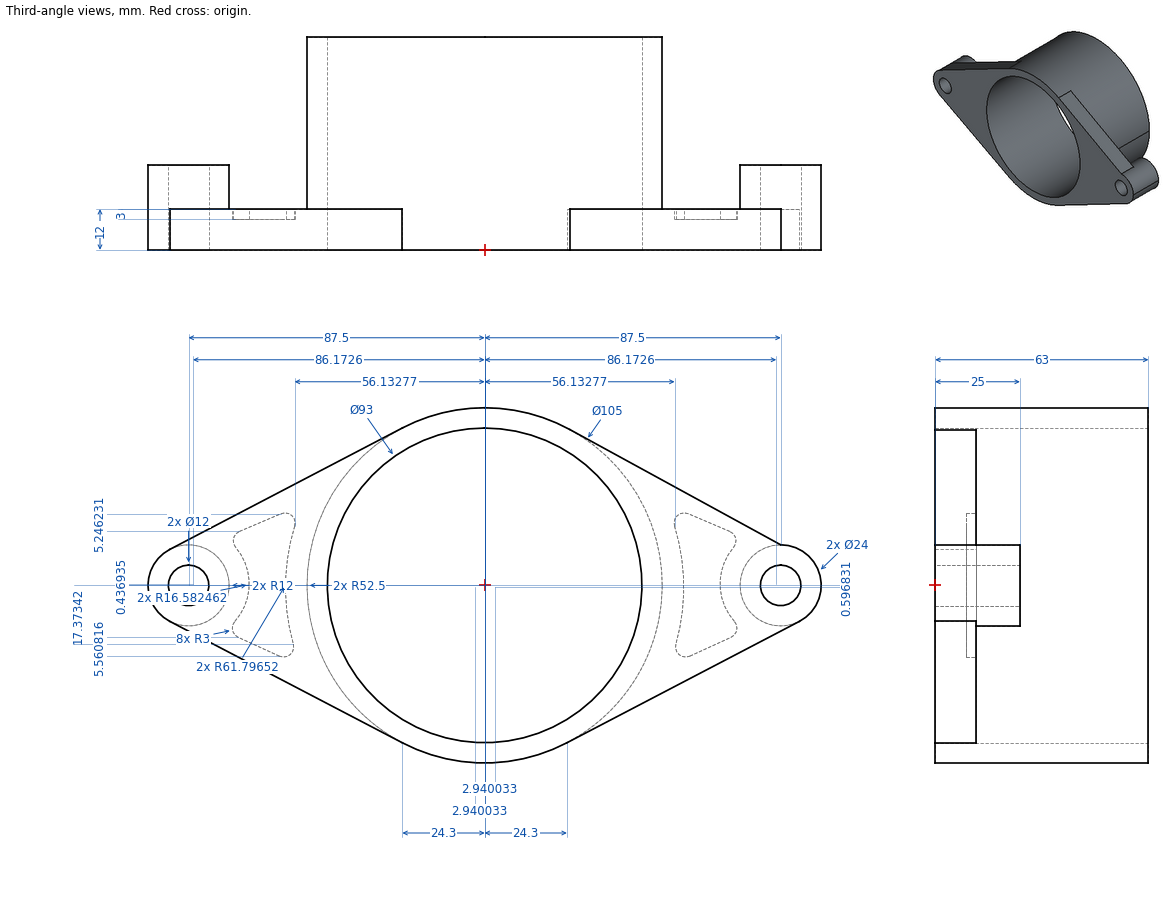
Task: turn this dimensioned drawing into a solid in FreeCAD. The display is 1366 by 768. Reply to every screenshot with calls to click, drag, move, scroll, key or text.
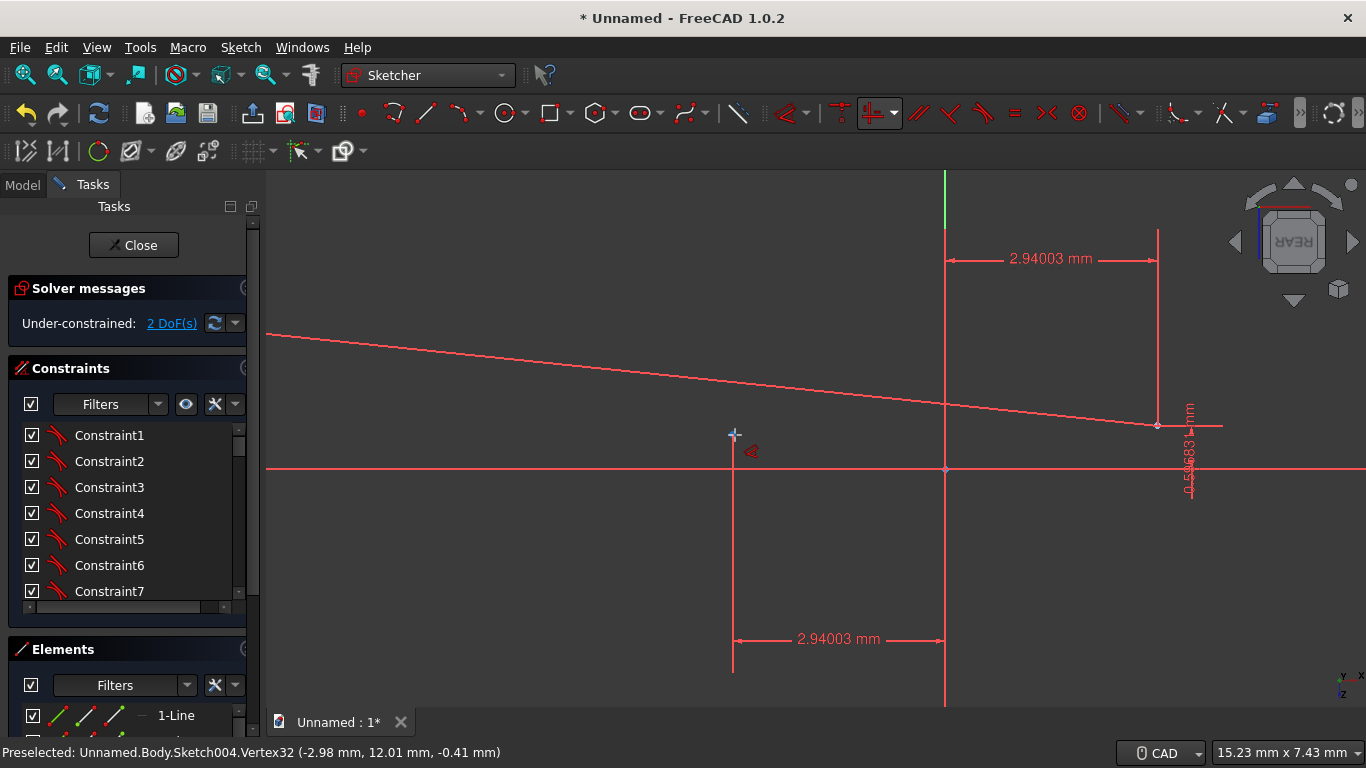
click(733, 434)
click(699, 452)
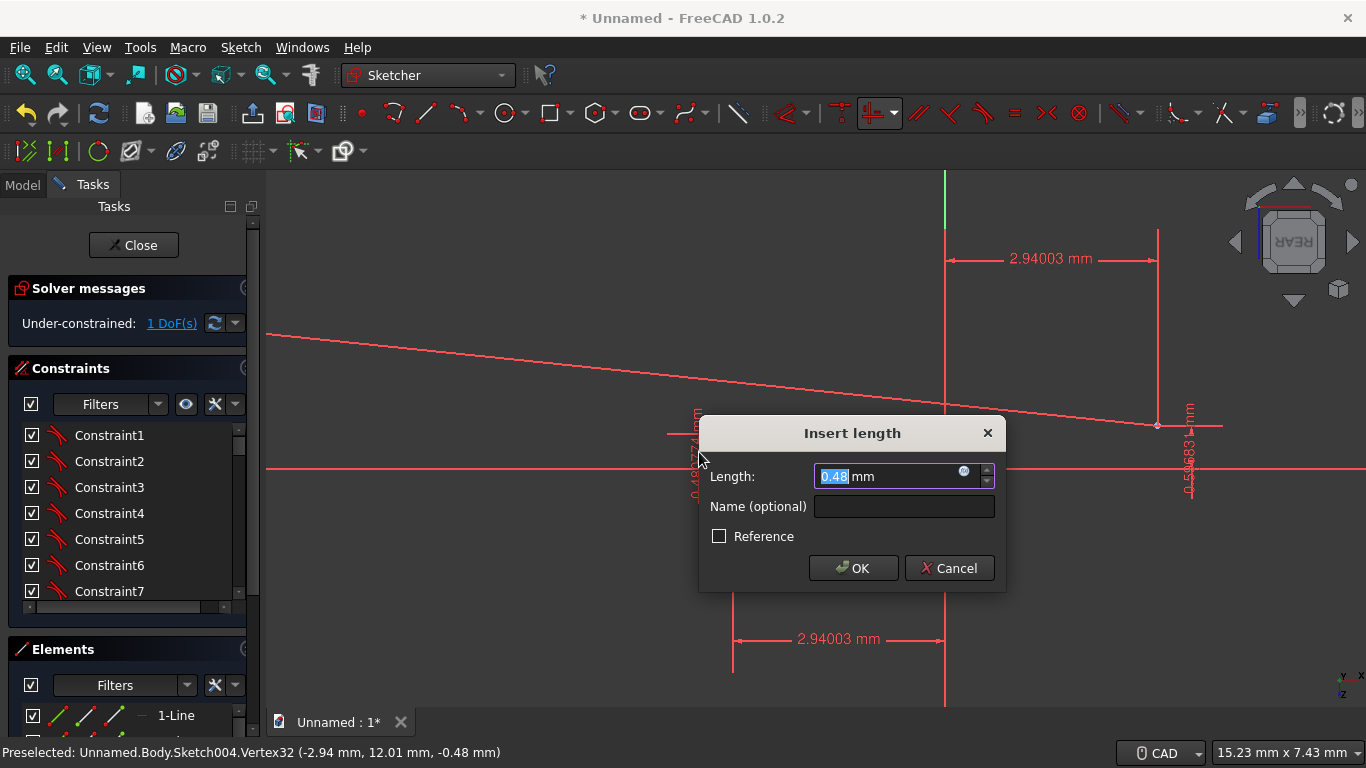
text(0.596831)
key(Return)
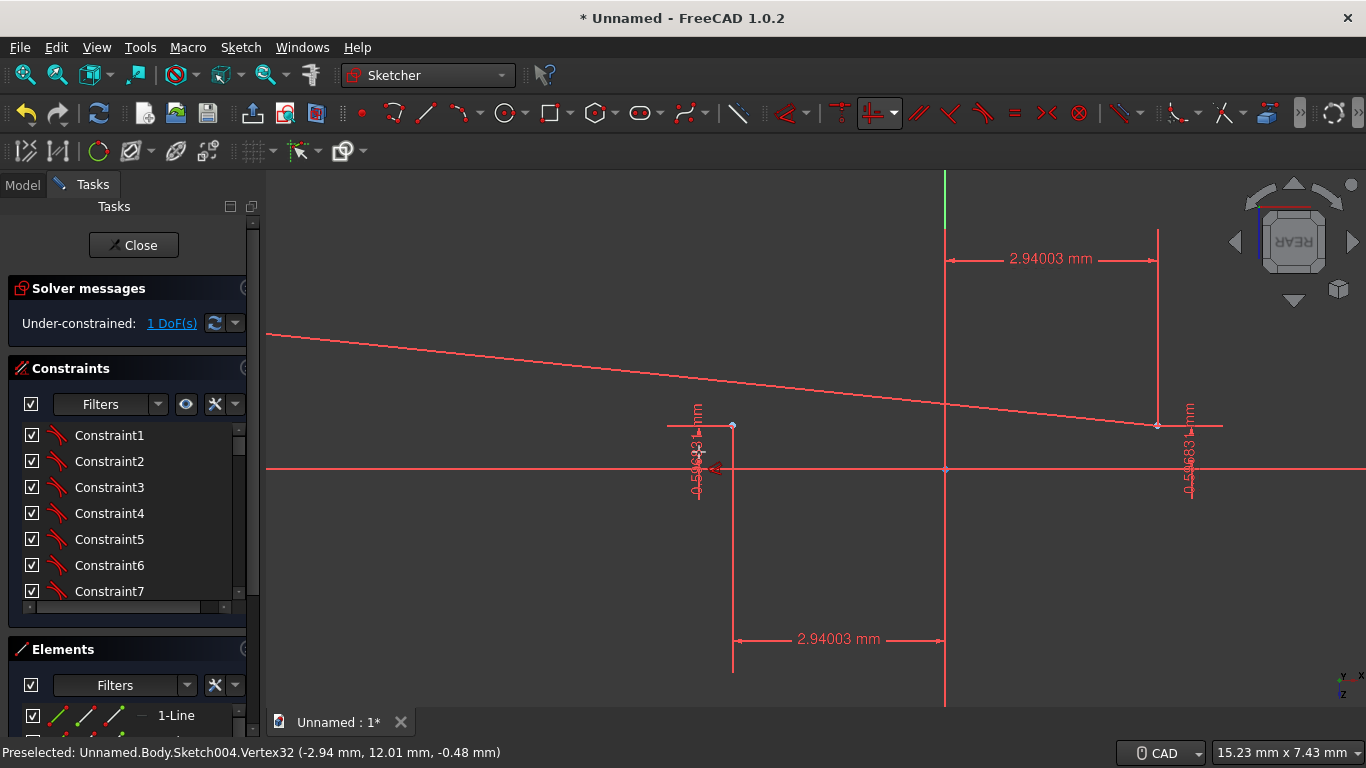
scroll(735, 436, down, 14)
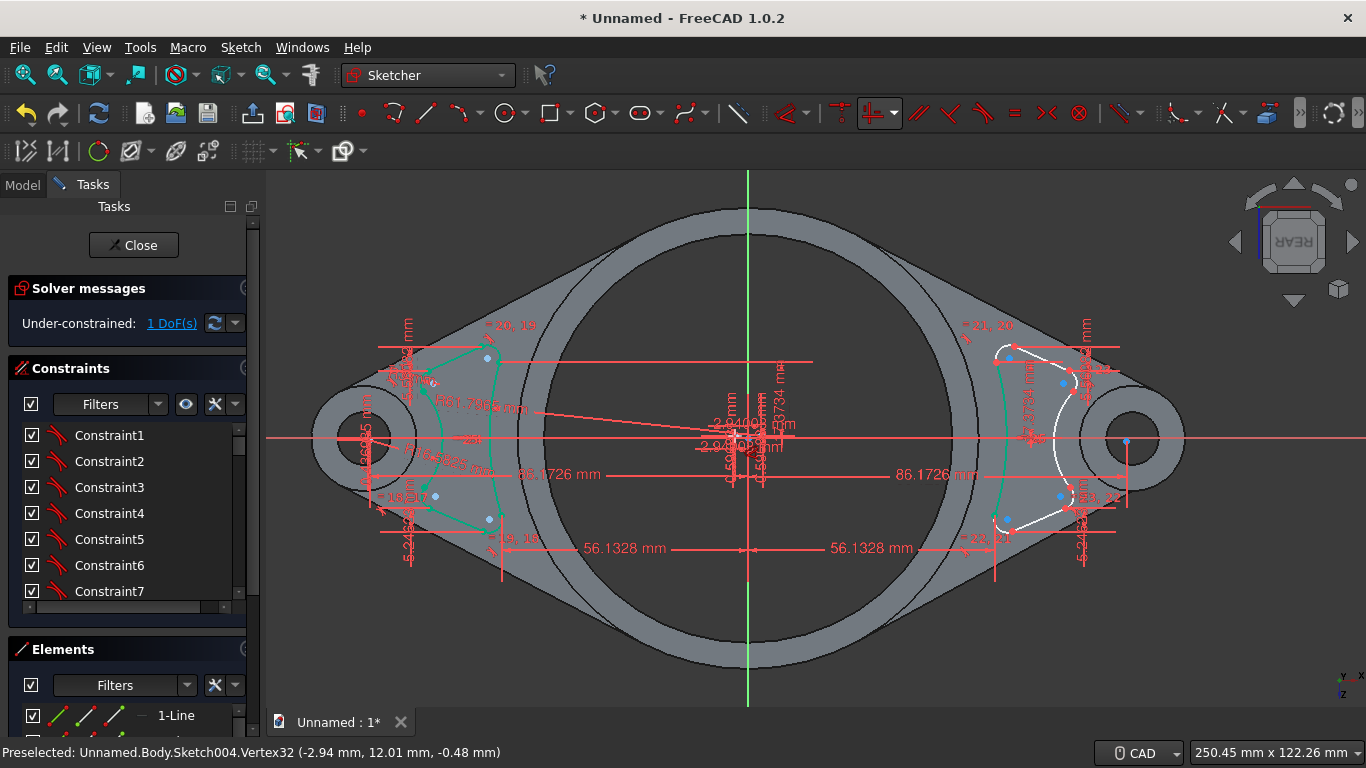
scroll(1127, 442, up, 16)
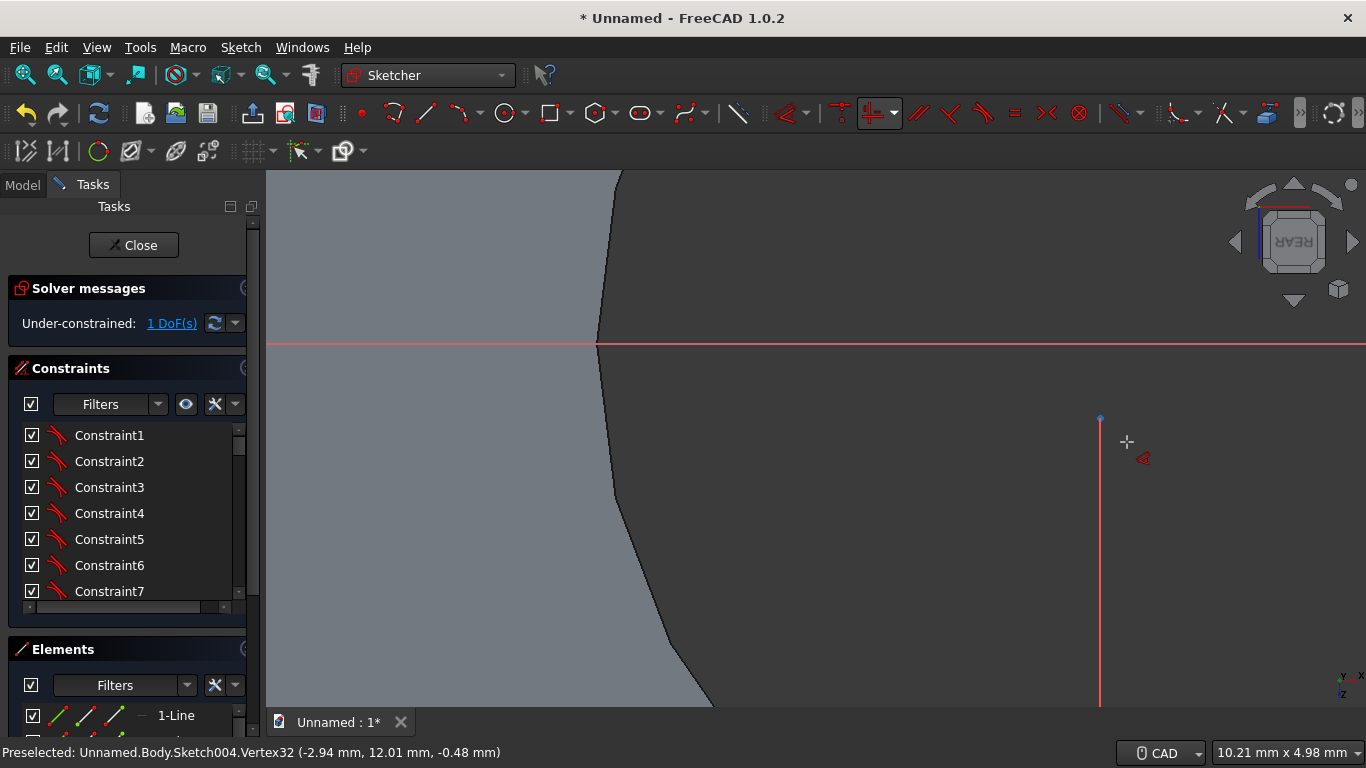
click(1100, 418)
click(1134, 381)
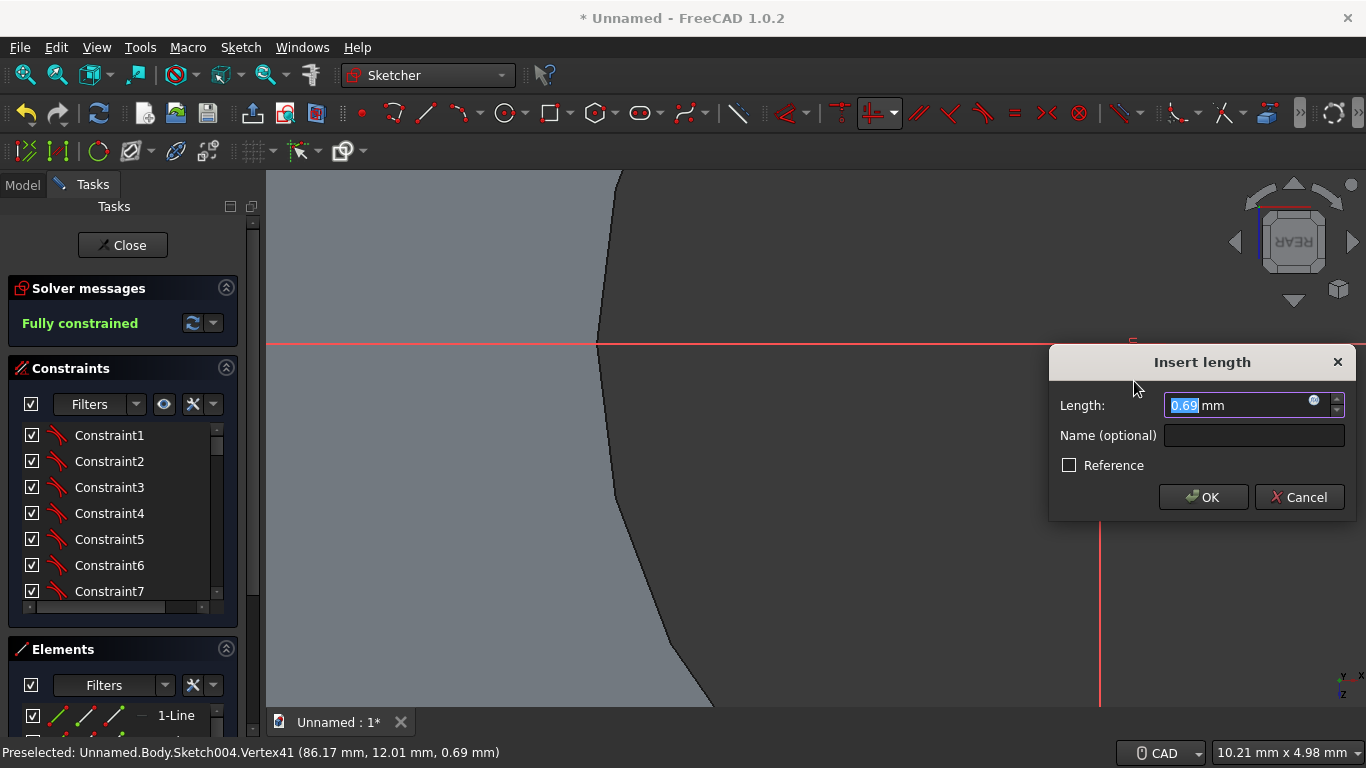
text(0.436935)
key(Return)
key(Escape)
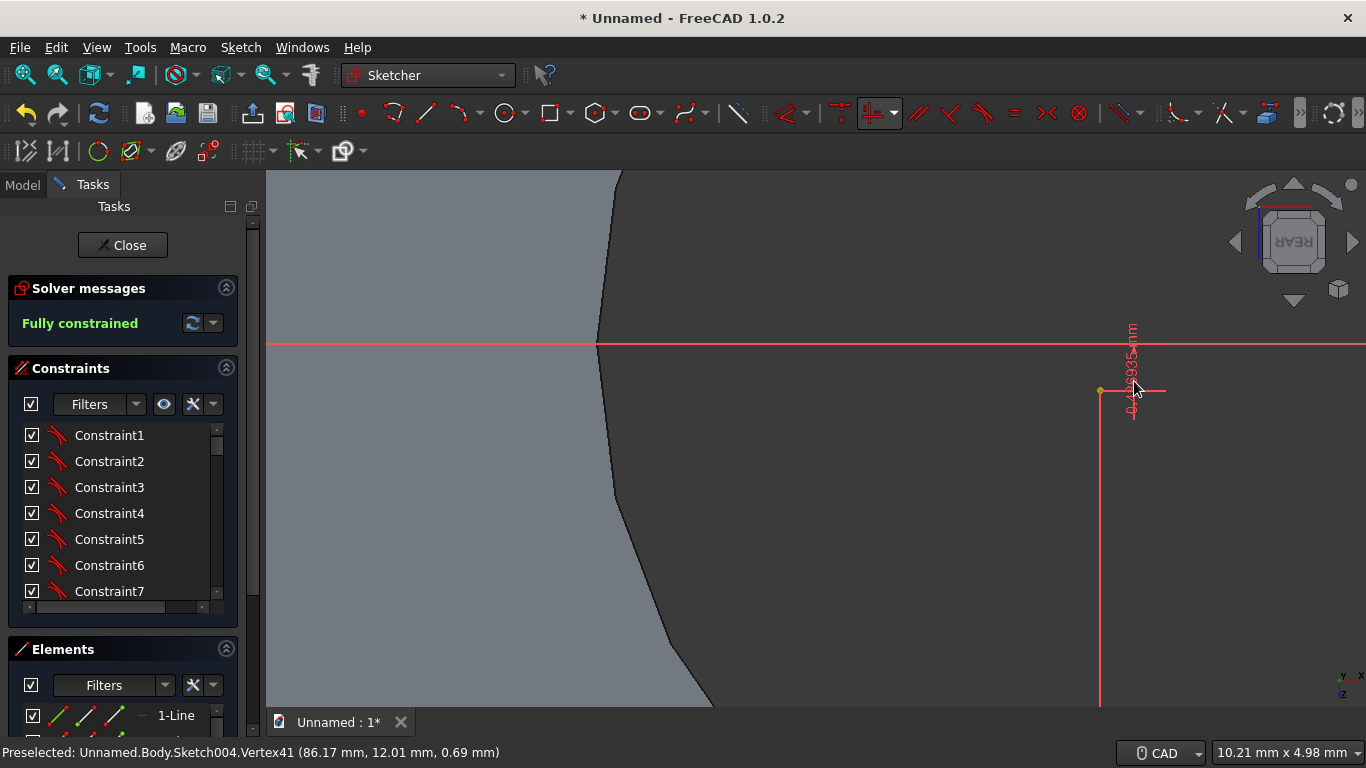
click(123, 245)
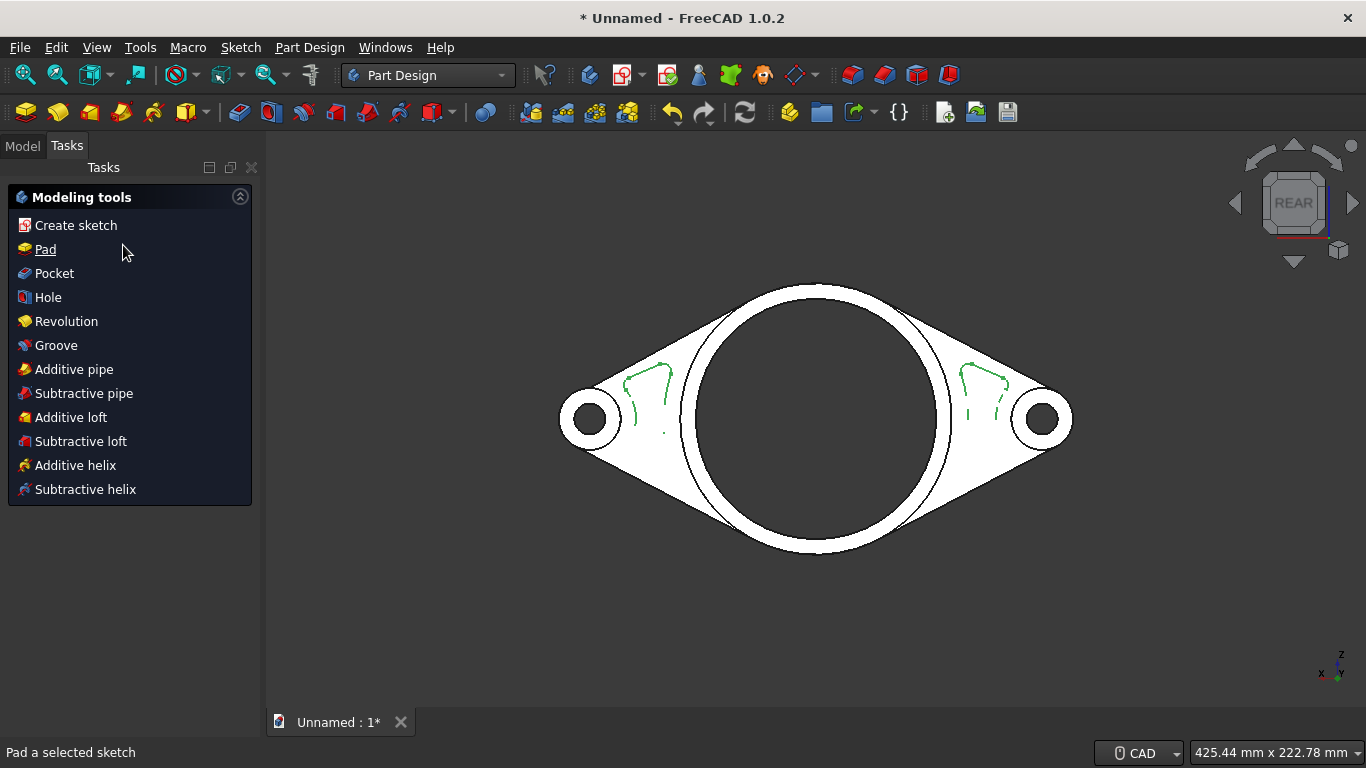
click(240, 112)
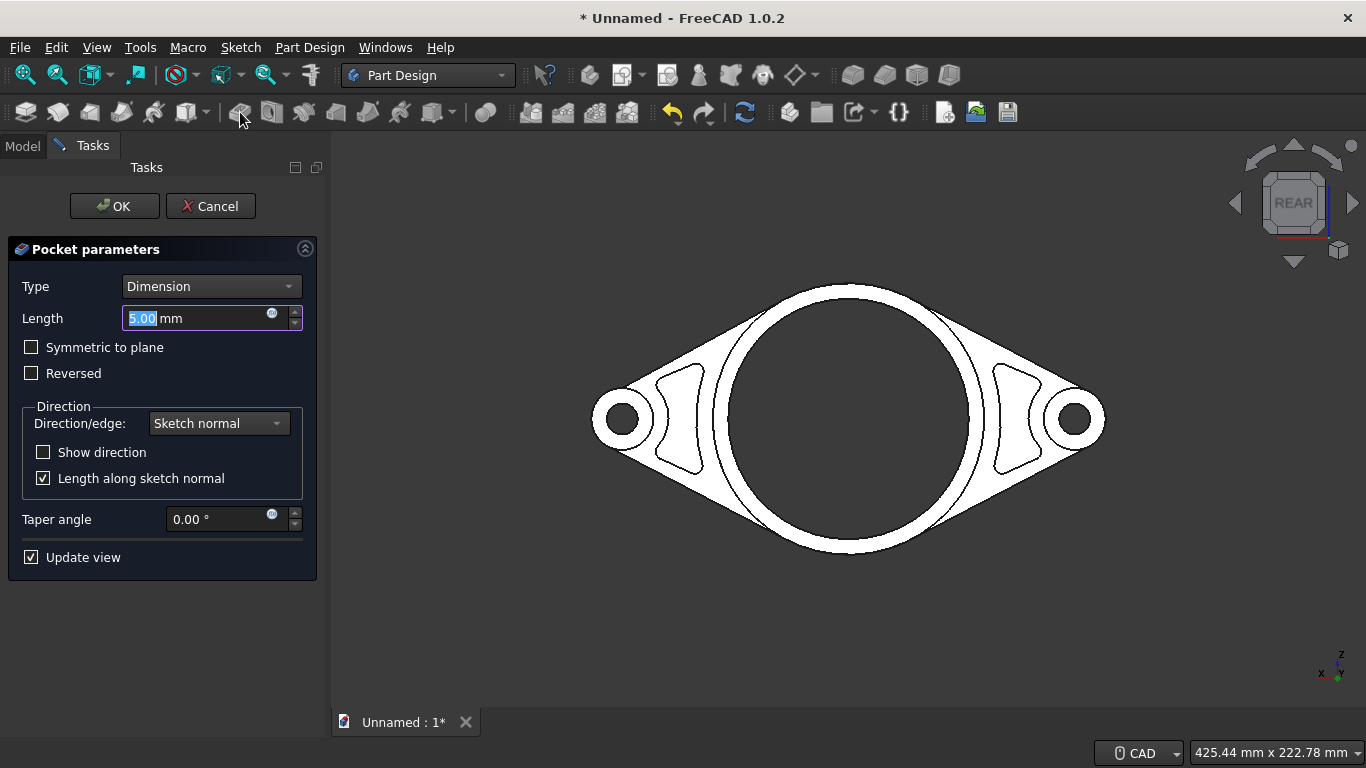
text(3)
key(Tab)